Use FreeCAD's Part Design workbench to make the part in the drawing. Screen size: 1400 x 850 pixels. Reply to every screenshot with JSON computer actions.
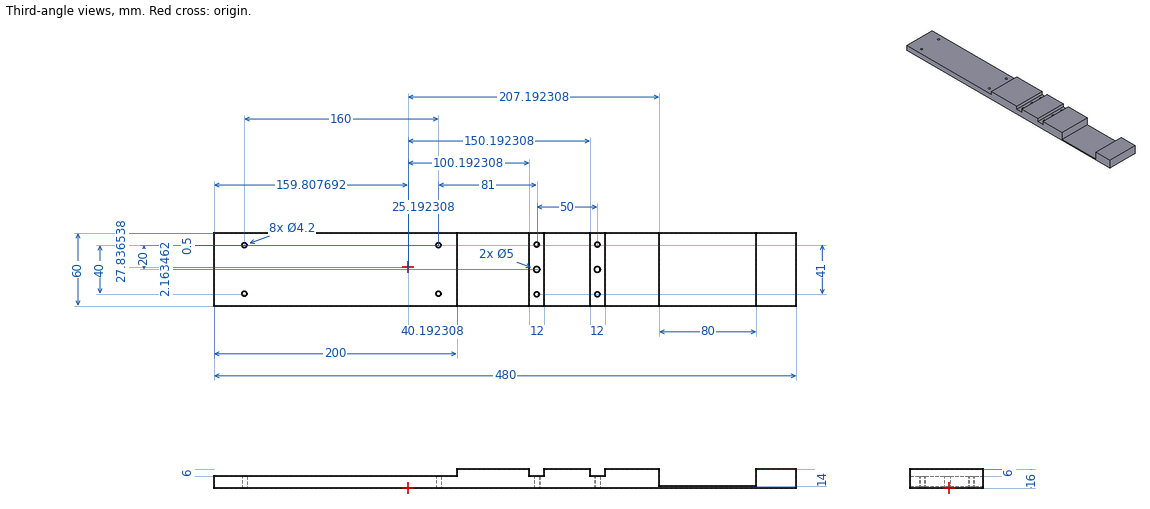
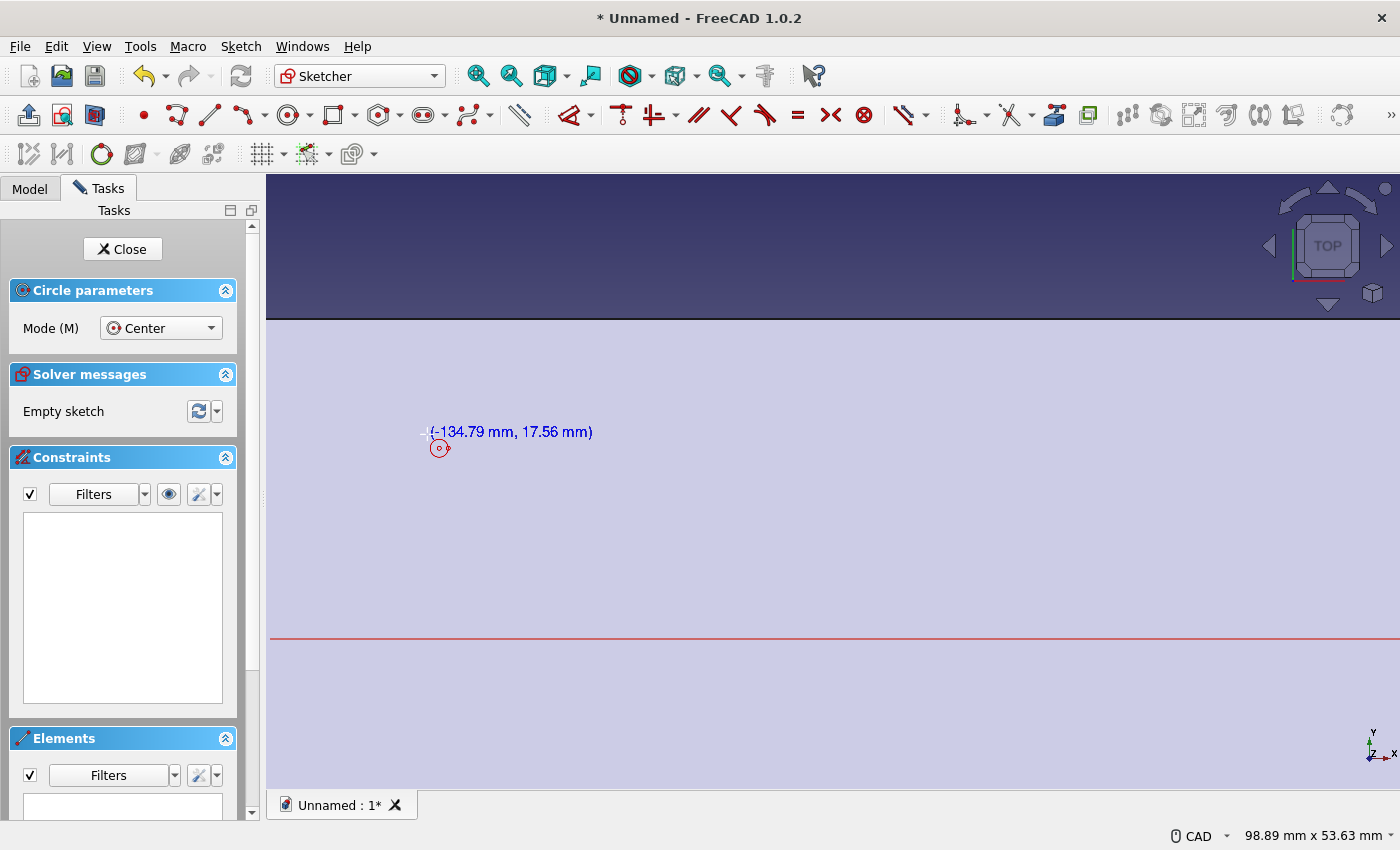
{"action": "scroll", "coordinate": [427, 435], "scroll_direction": "down", "scroll_amount": 8}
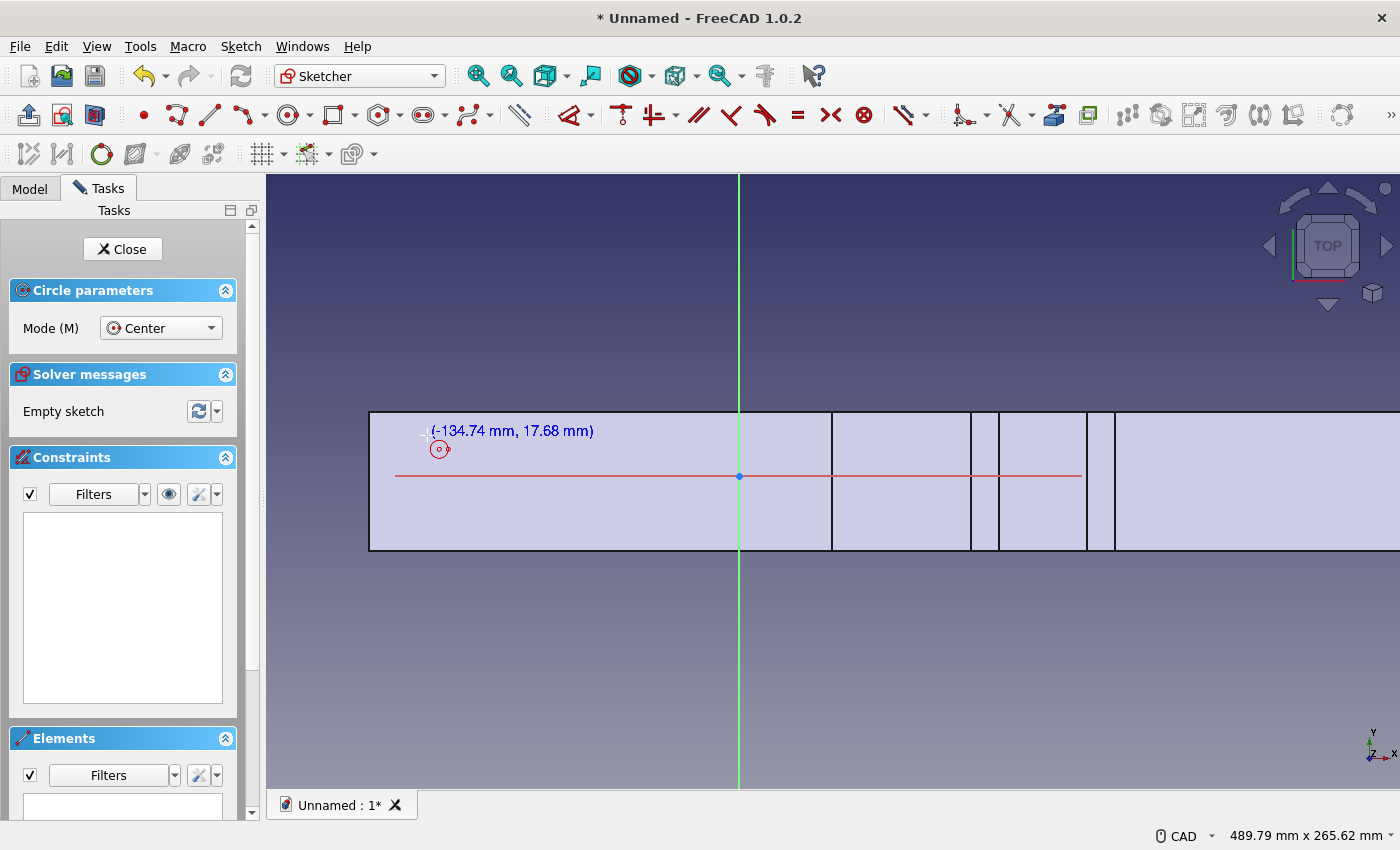
{"action": "left_click", "coordinate": [427, 435]}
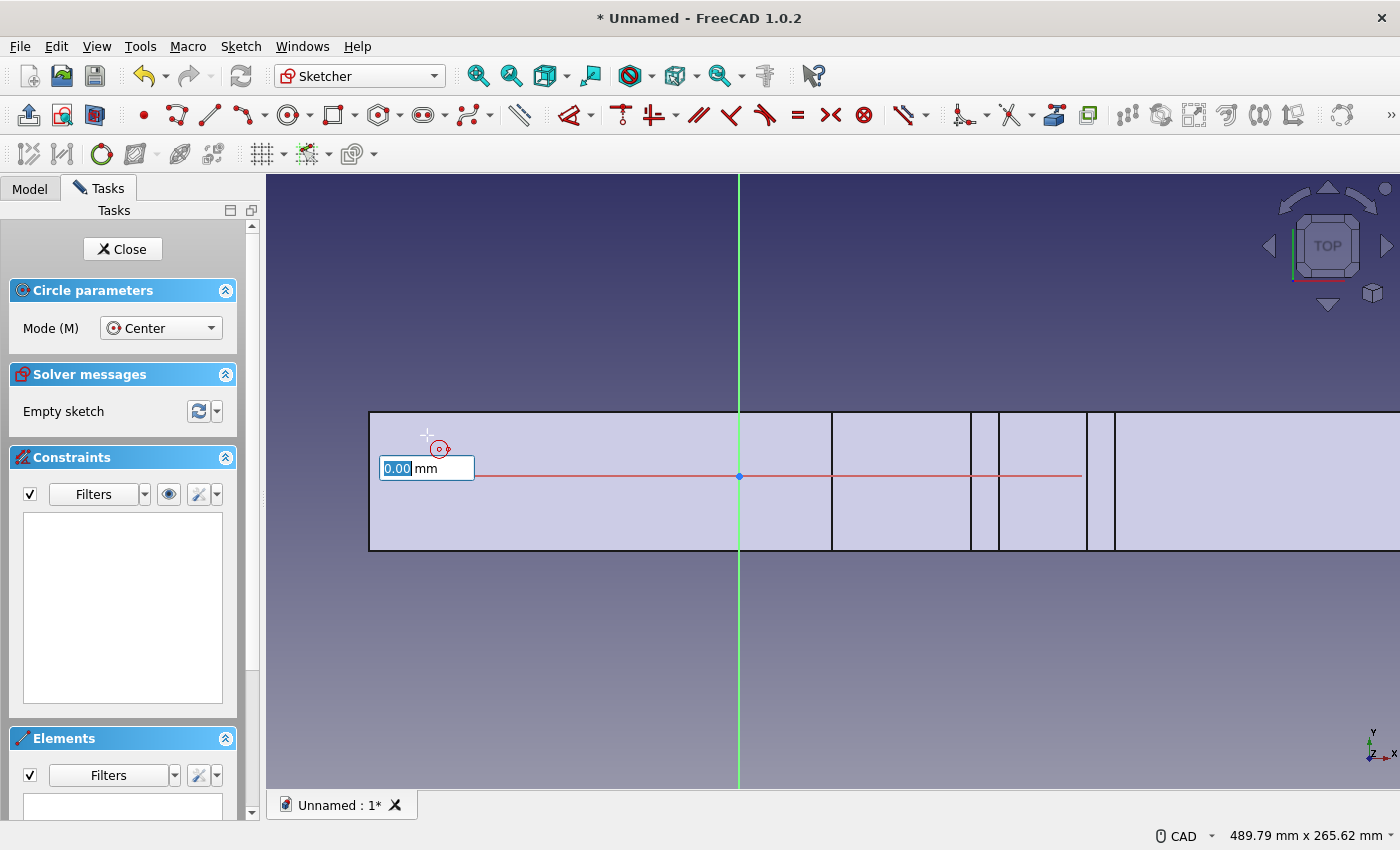
{"action": "scroll", "coordinate": [430, 432], "scroll_direction": "up", "scroll_amount": 6}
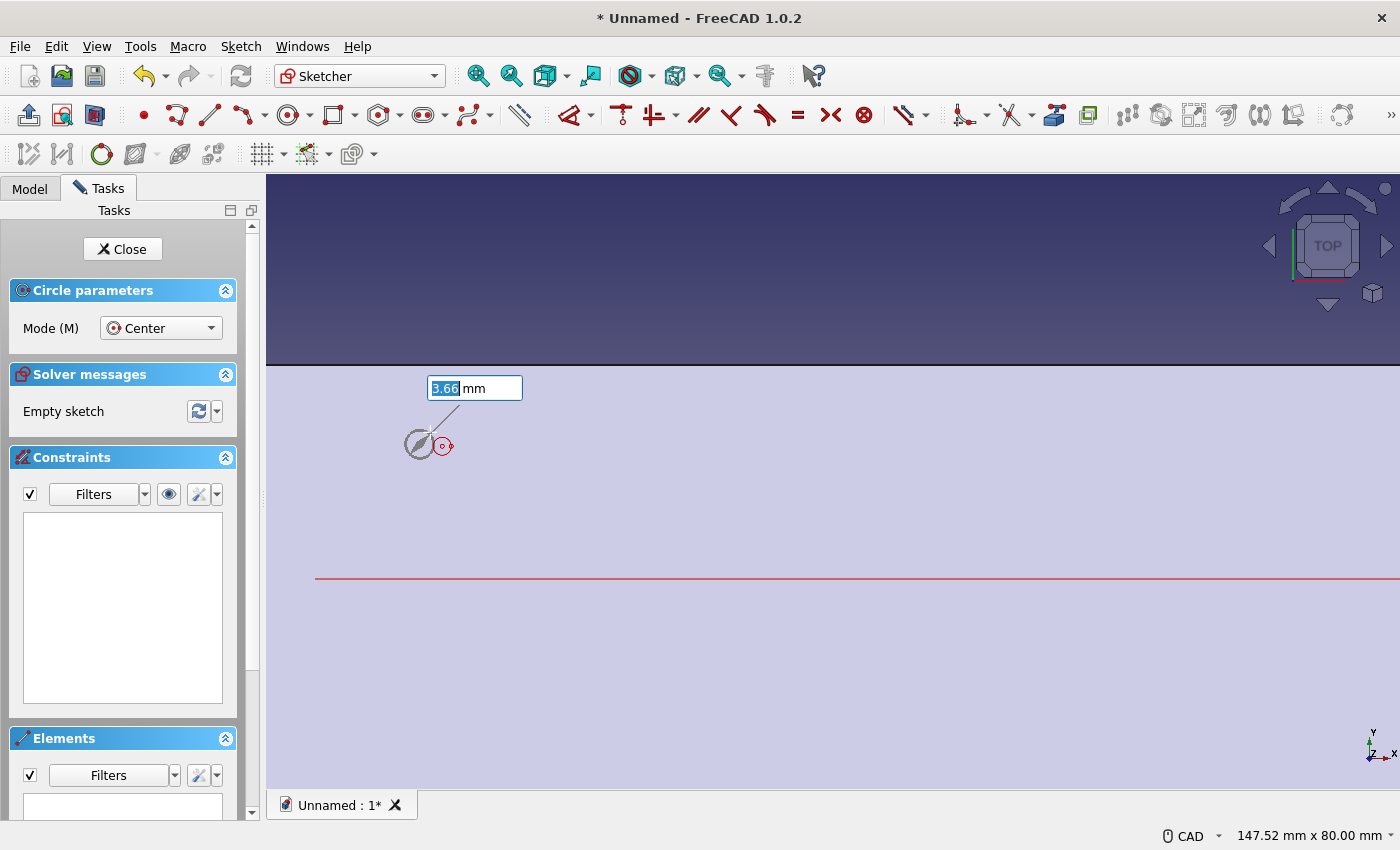
{"action": "left_click", "coordinate": [431, 430]}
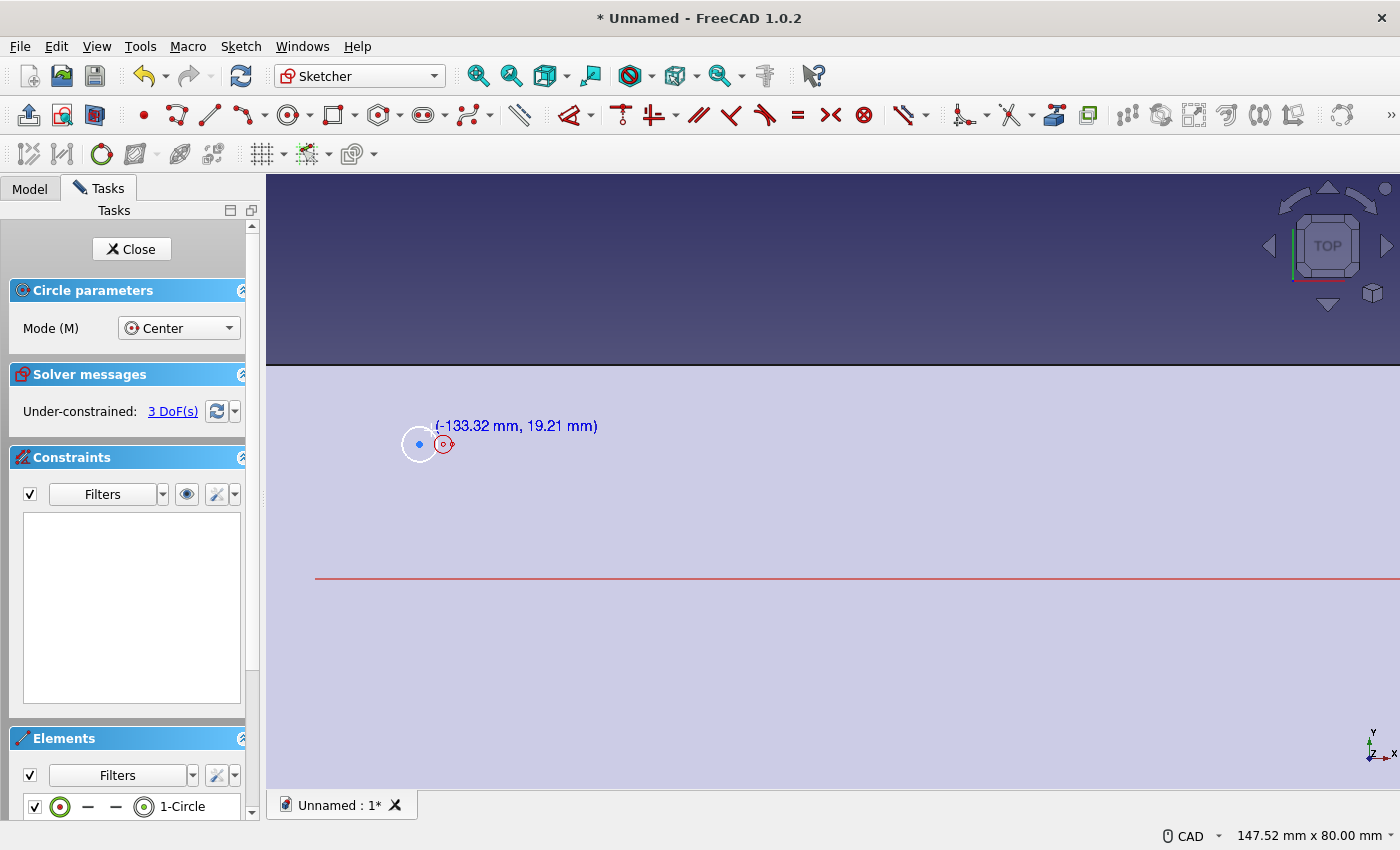
{"action": "scroll", "coordinate": [420, 749], "scroll_direction": "up", "scroll_amount": 2}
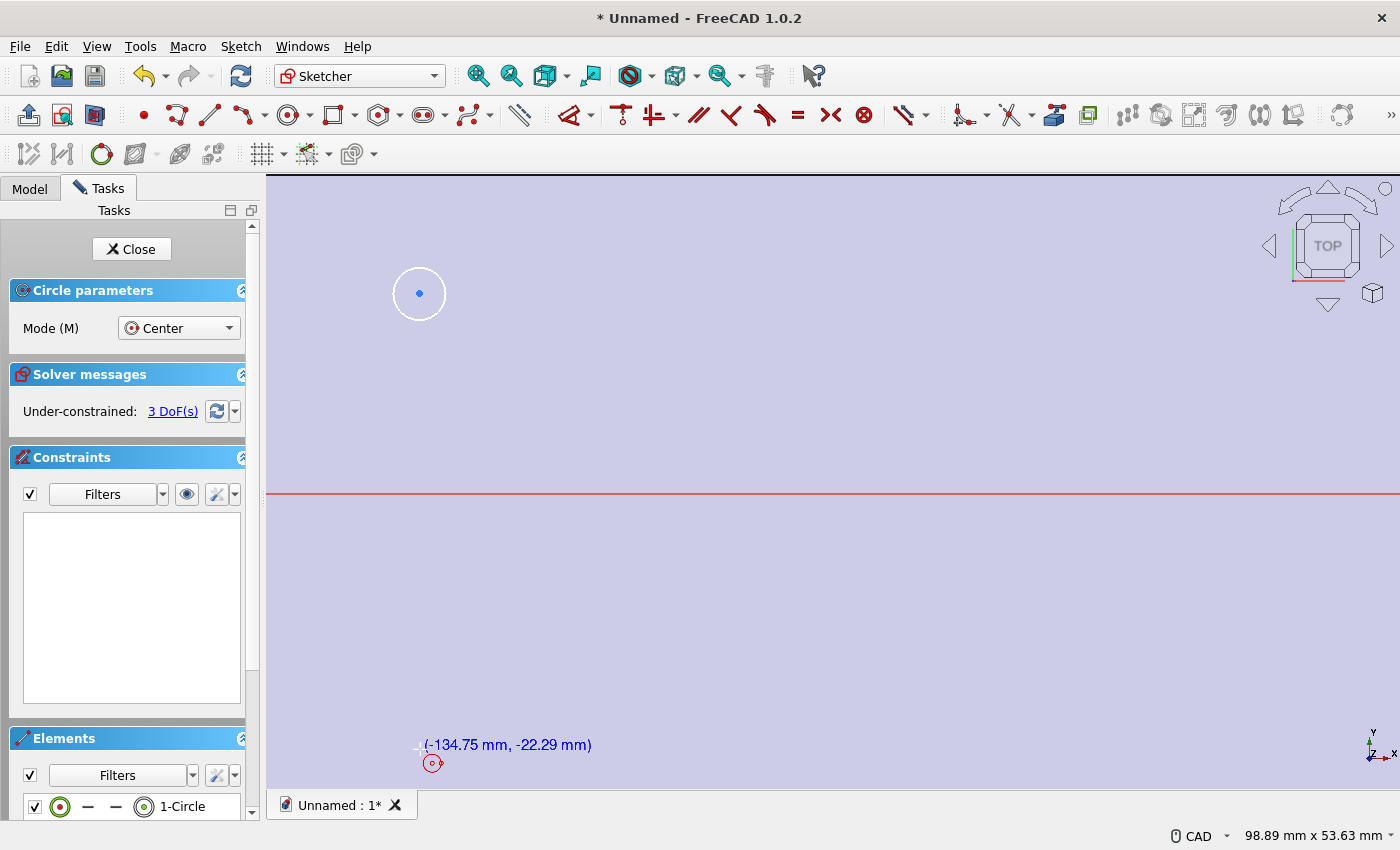
{"action": "scroll", "coordinate": [429, 472], "scroll_direction": "down", "scroll_amount": 8}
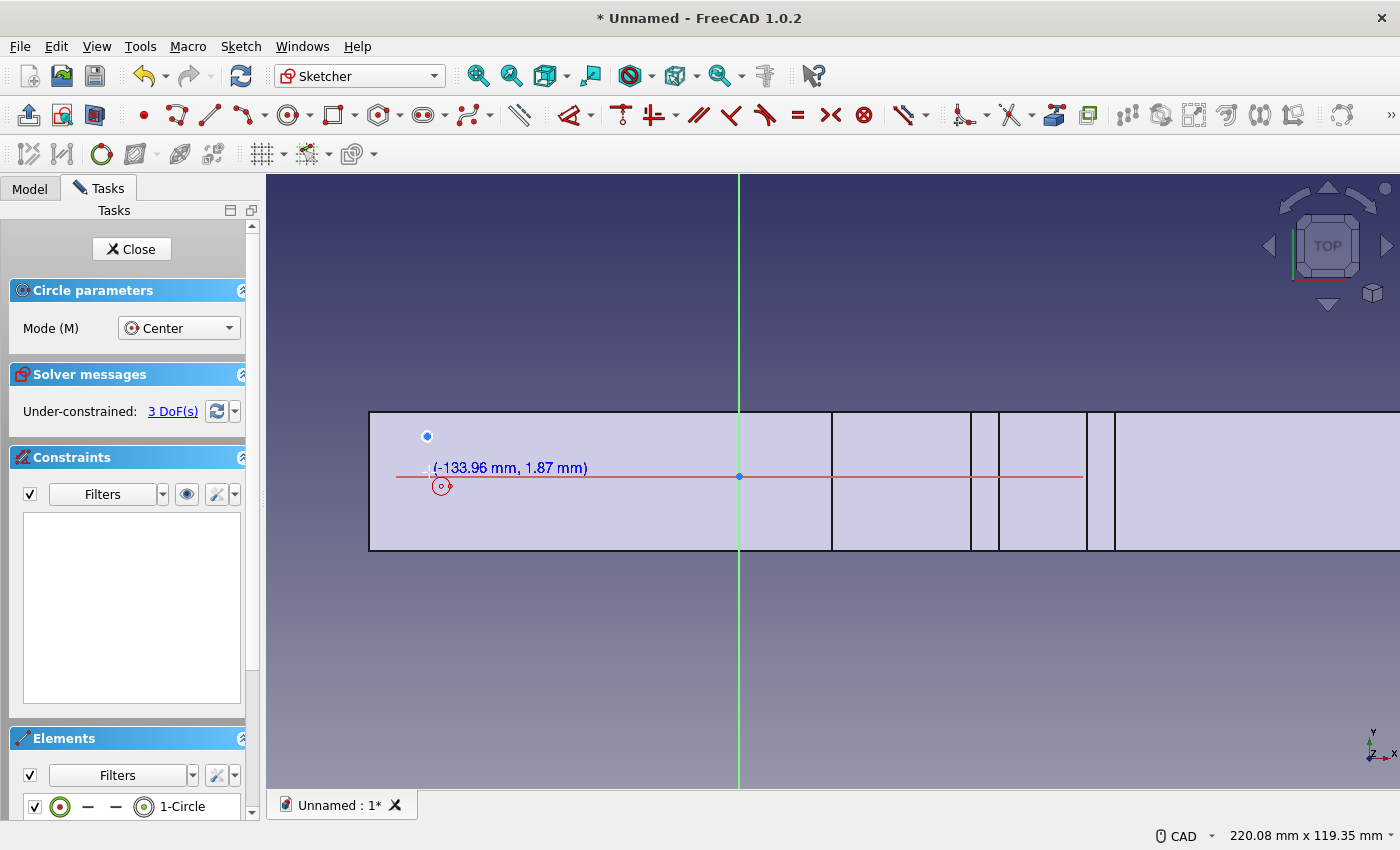
{"action": "left_click", "coordinate": [427, 528]}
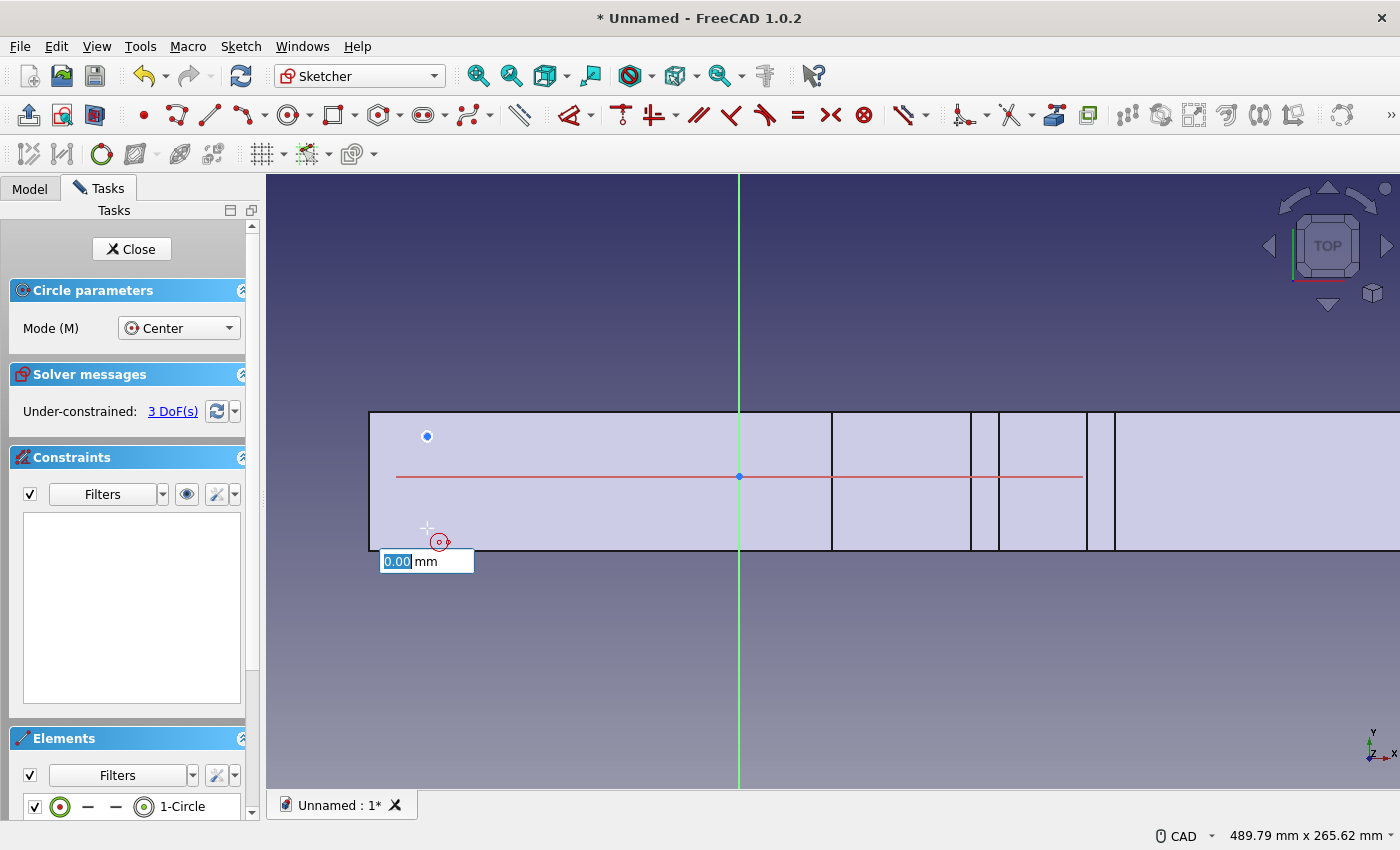
{"action": "scroll", "coordinate": [431, 525], "scroll_direction": "up", "scroll_amount": 6}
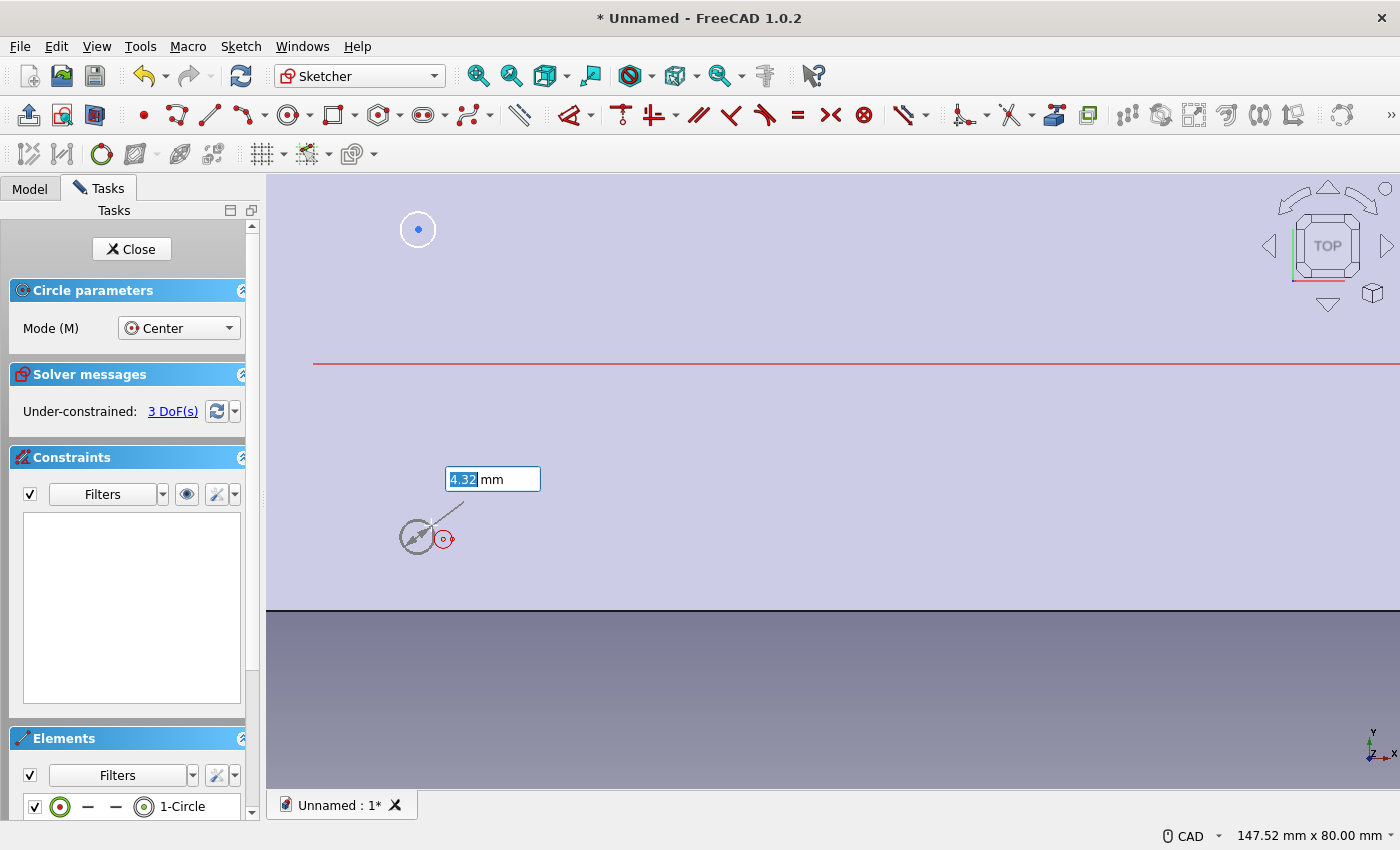
{"action": "left_click", "coordinate": [429, 523]}